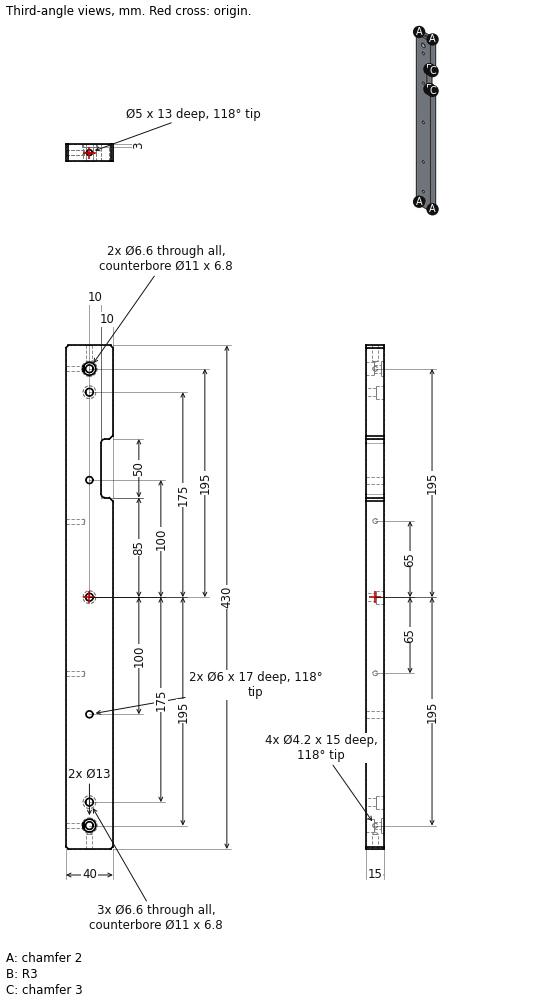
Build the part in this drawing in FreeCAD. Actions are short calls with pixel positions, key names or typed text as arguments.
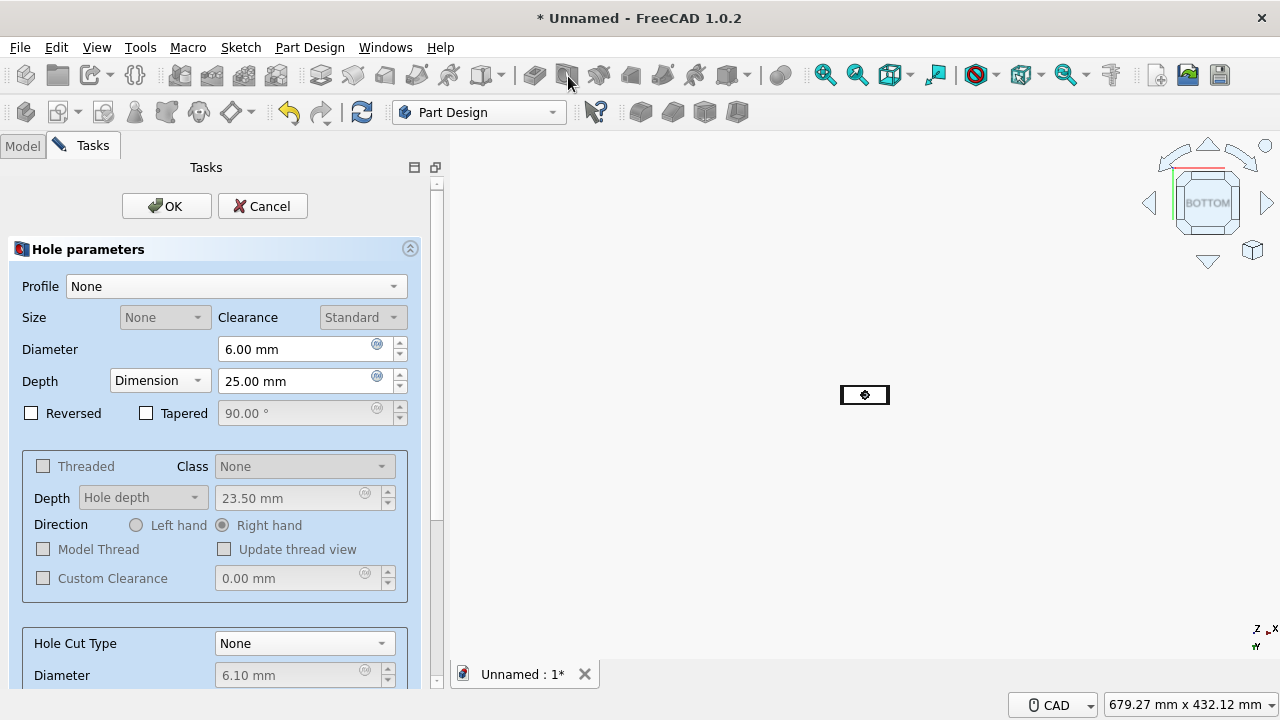
triple_click(305, 349)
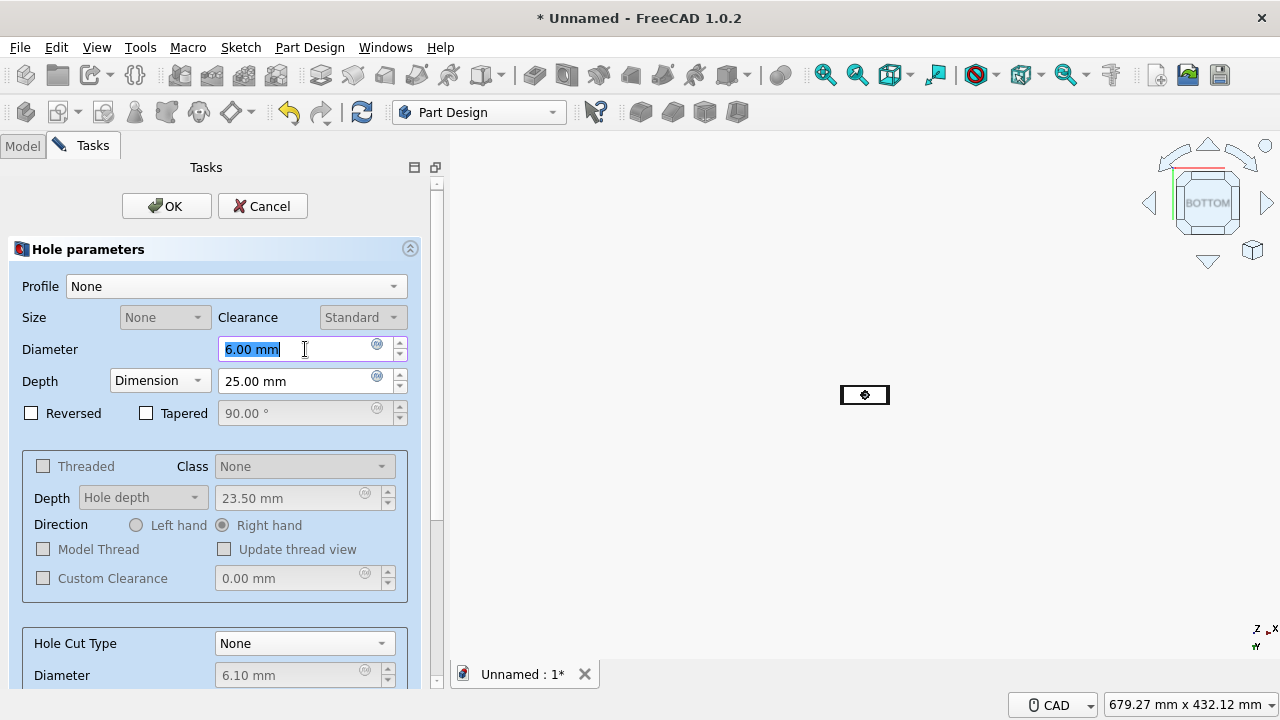
text(5)
key(Tab)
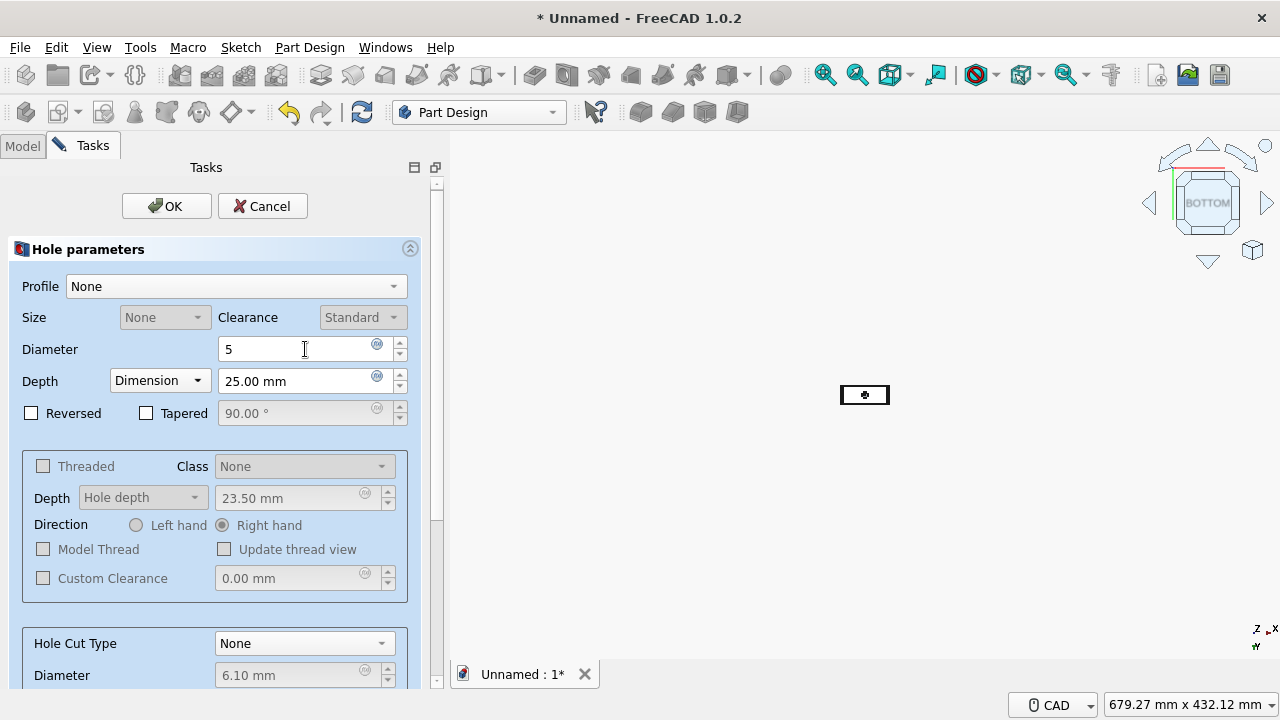
triple_click(305, 381)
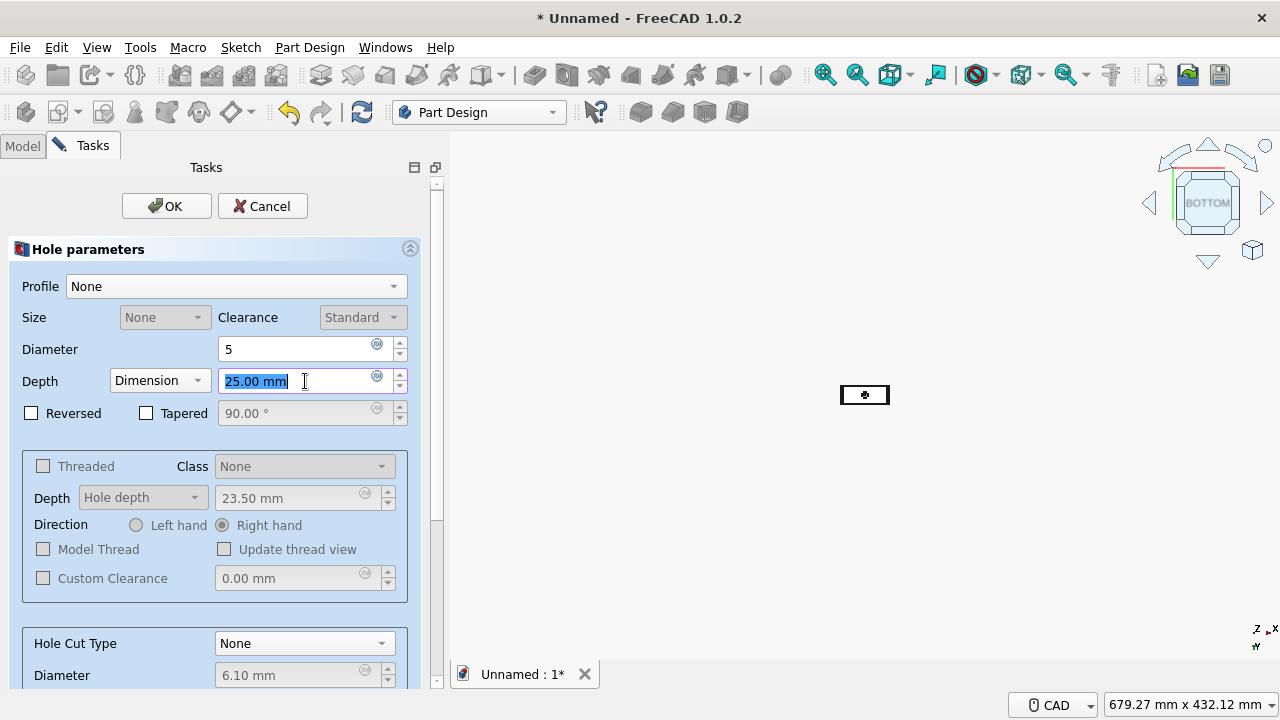
text(13)
key(Tab)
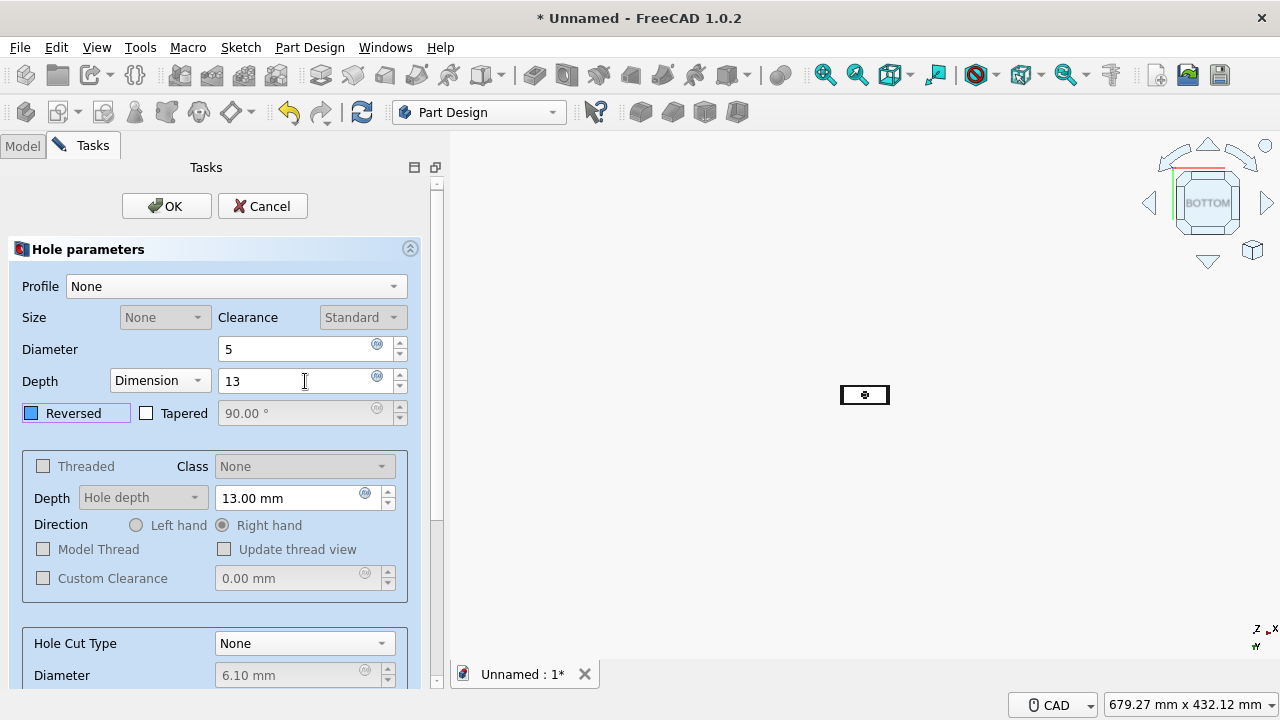
click(167, 206)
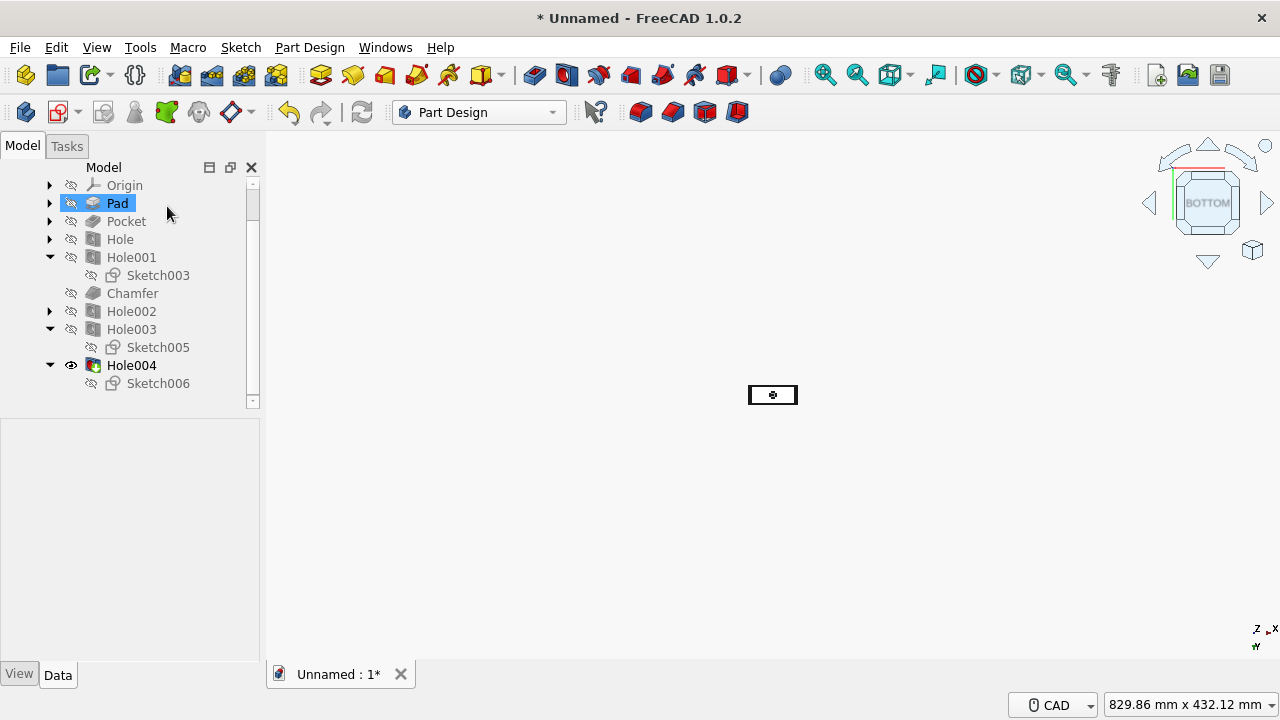
click(826, 76)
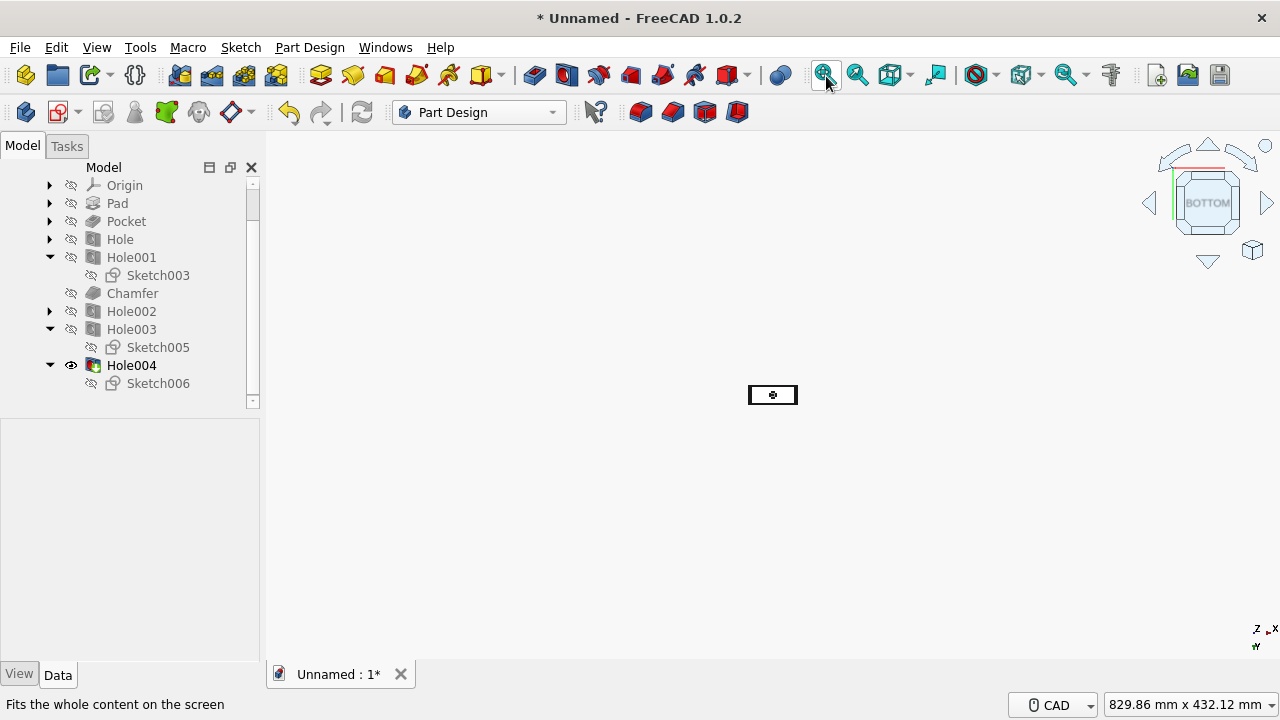
key(0)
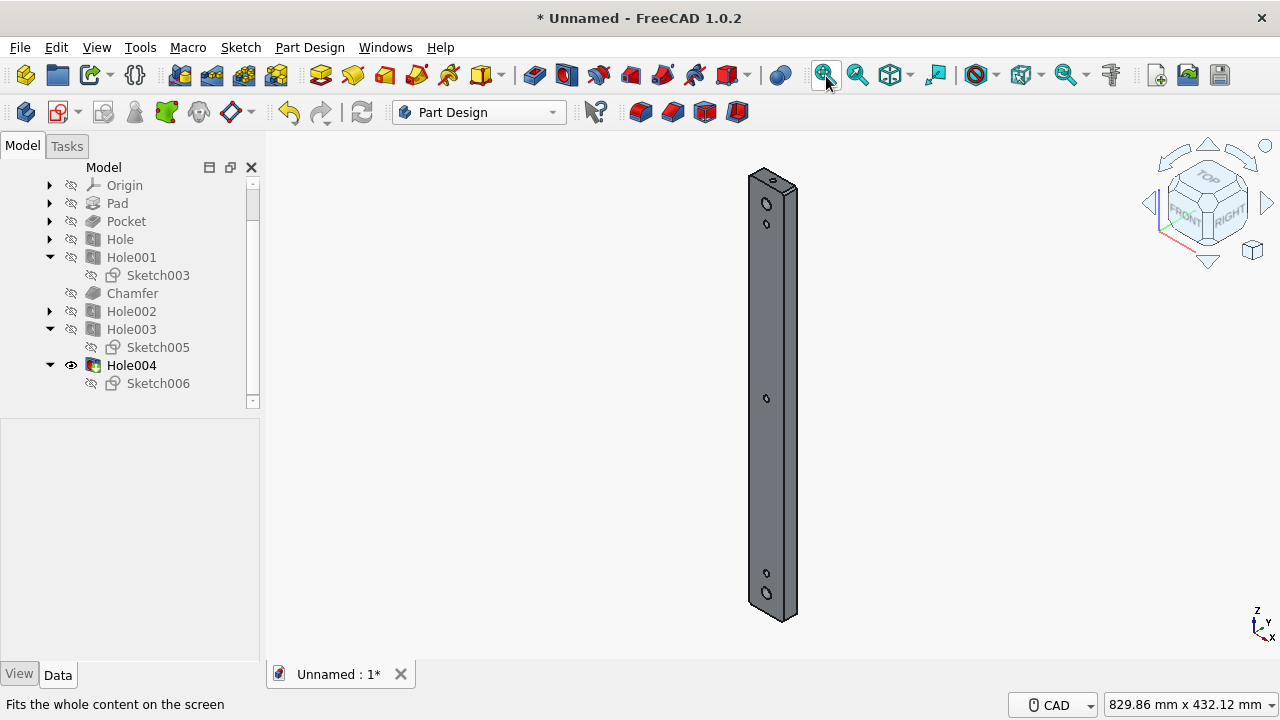
click(767, 275)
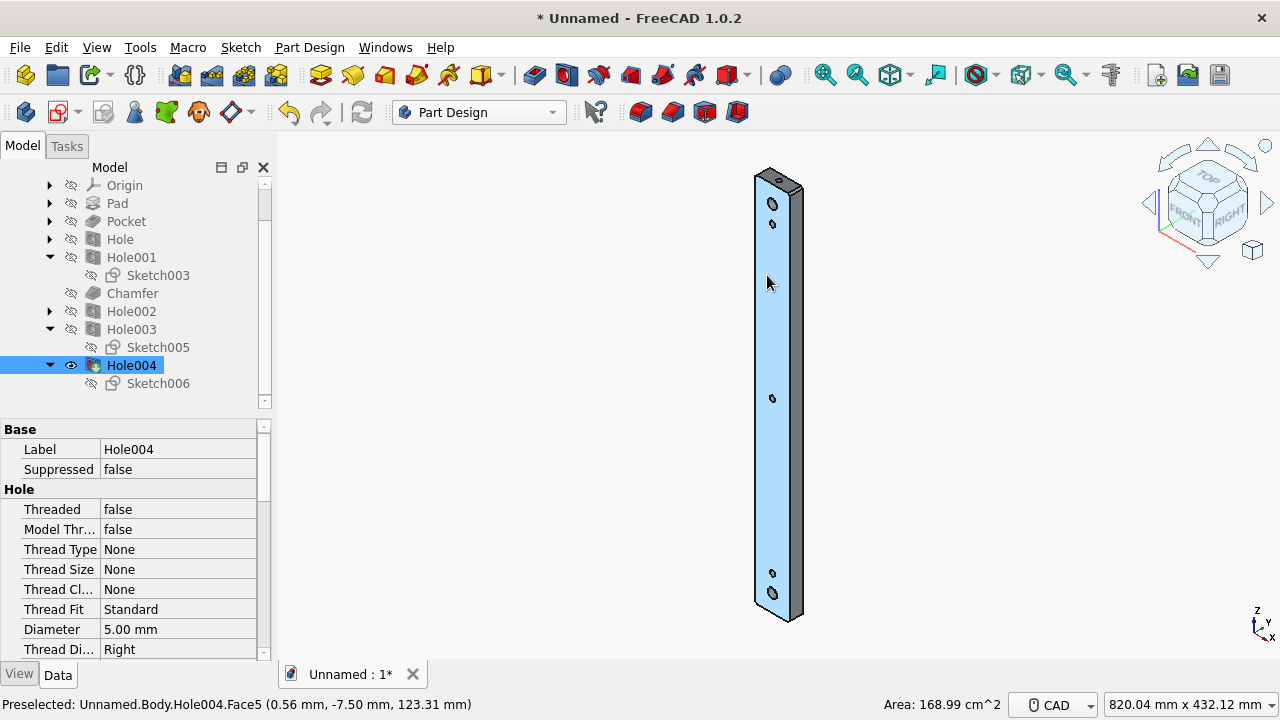
click(58, 112)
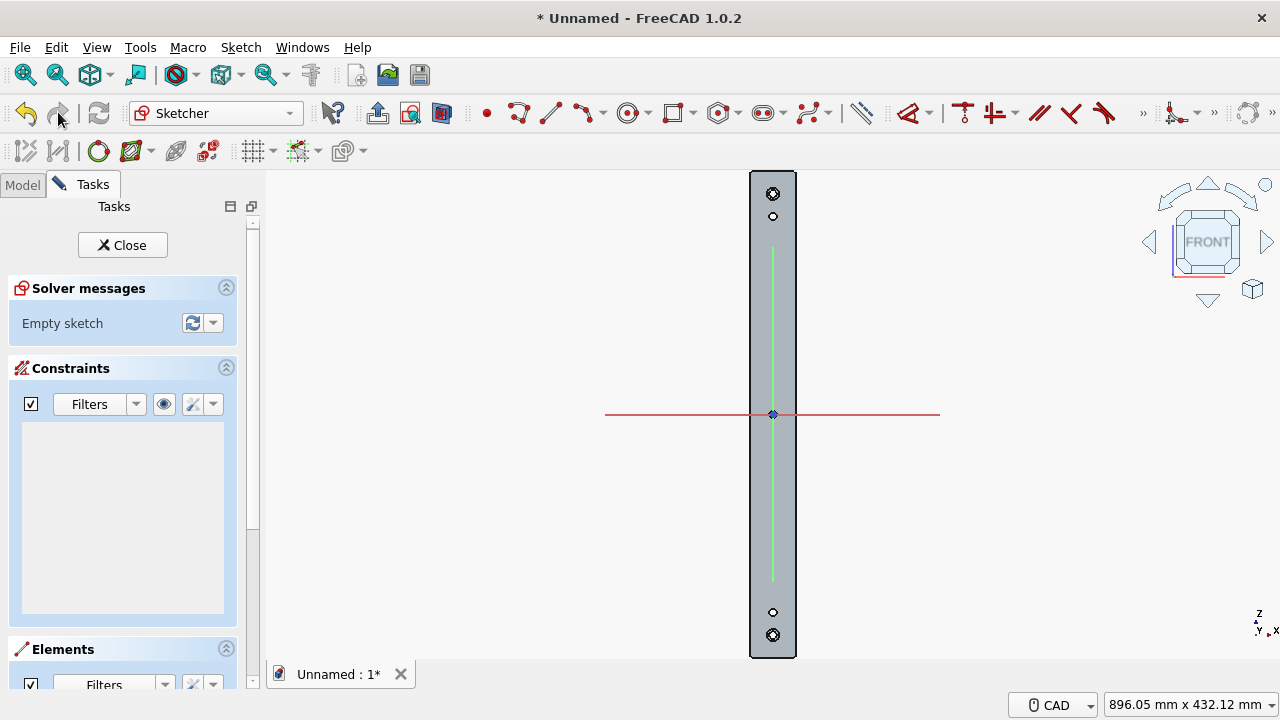
click(628, 114)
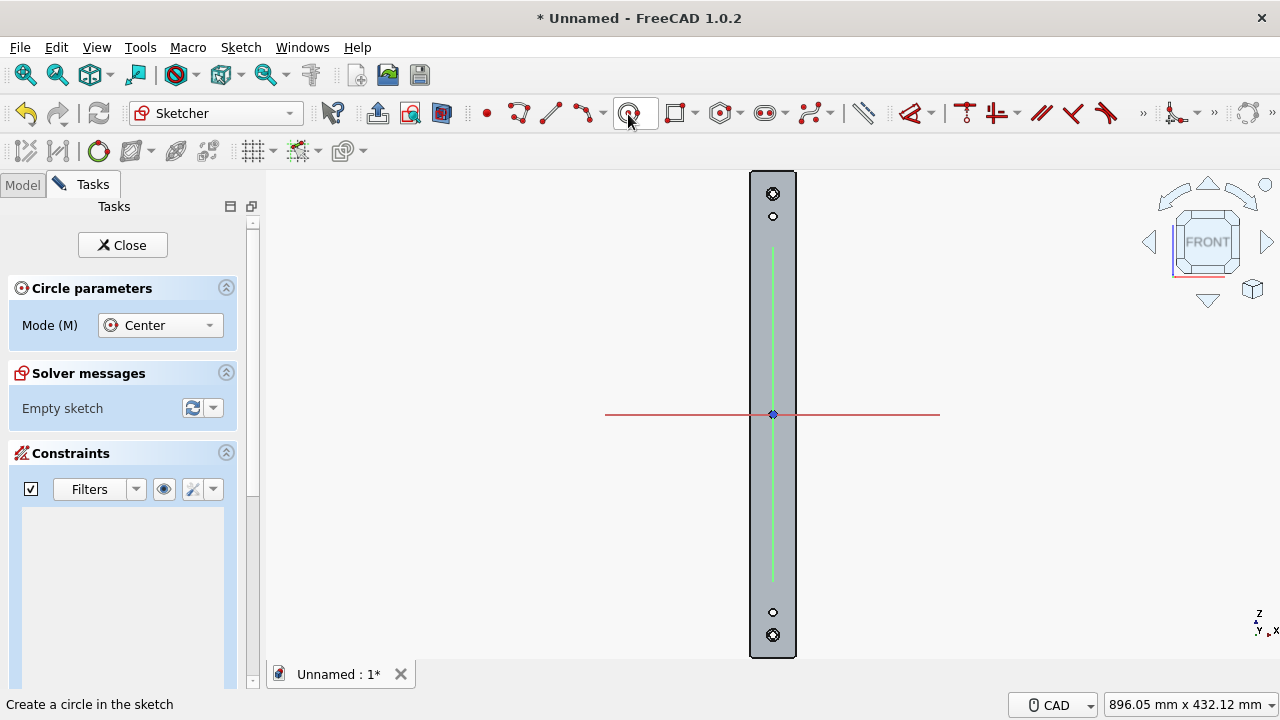
scroll(773, 528, up, 10)